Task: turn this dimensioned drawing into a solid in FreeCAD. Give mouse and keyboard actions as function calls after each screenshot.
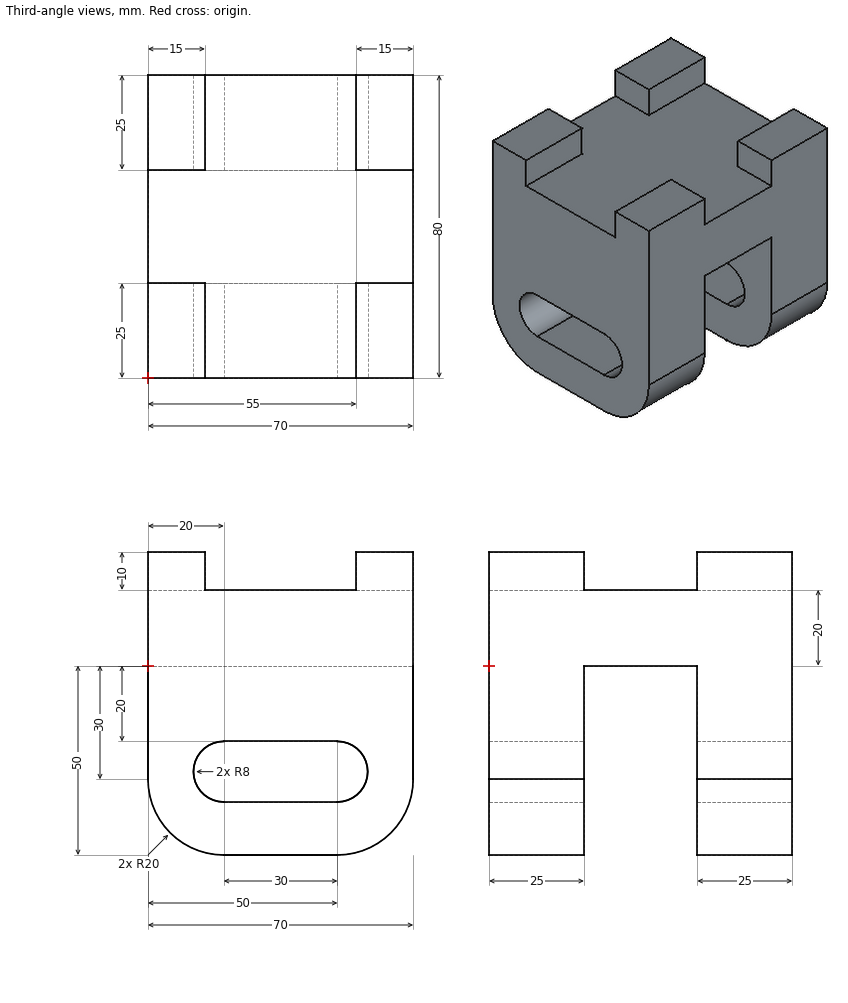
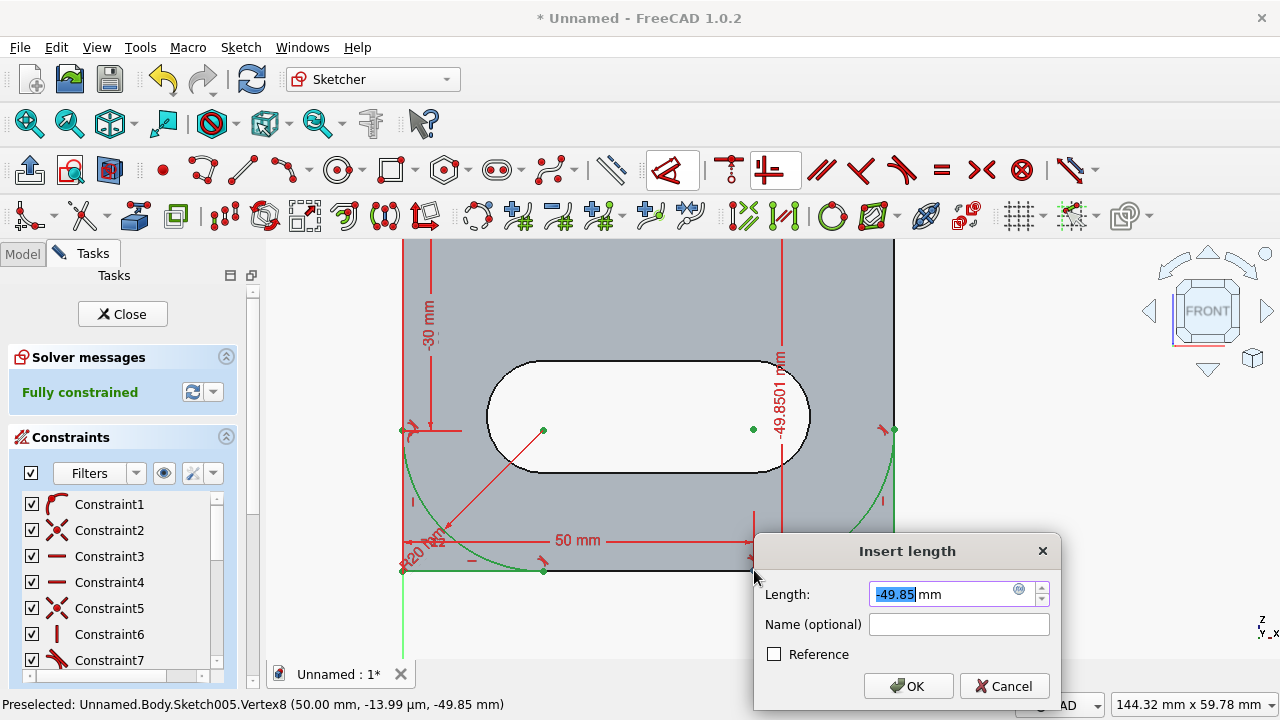
text(-50)
key(Return)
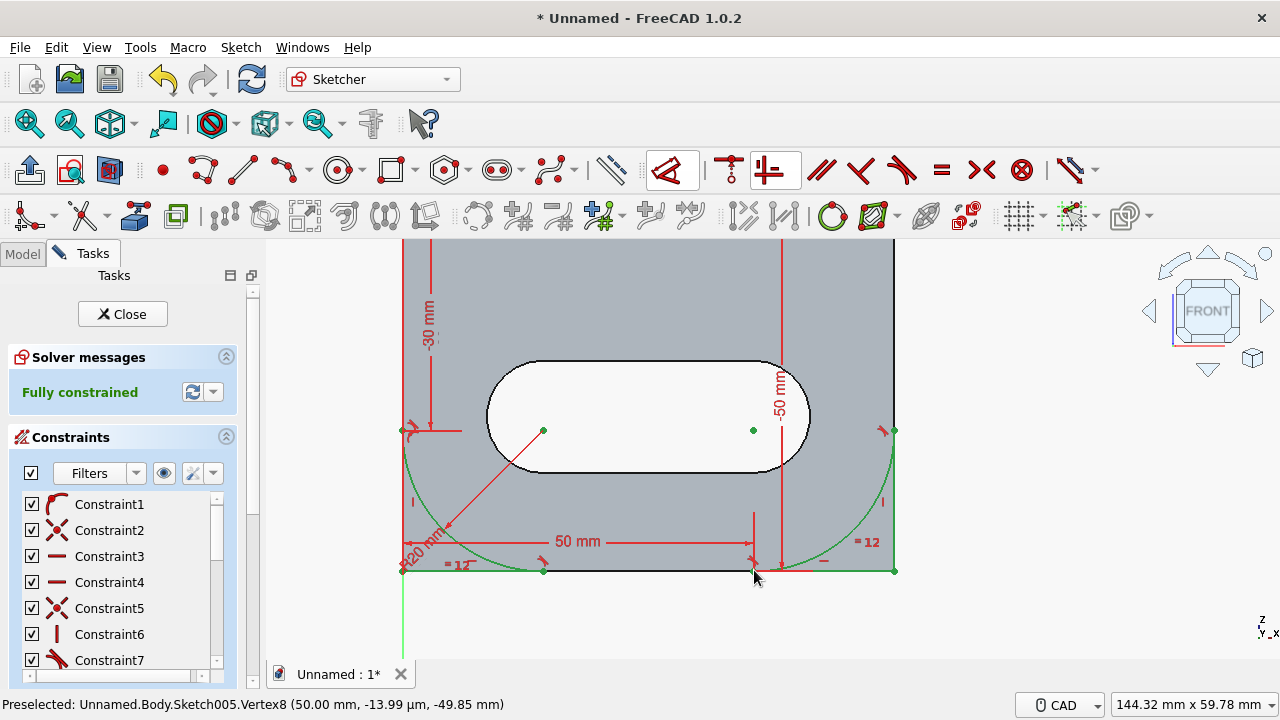
click(123, 314)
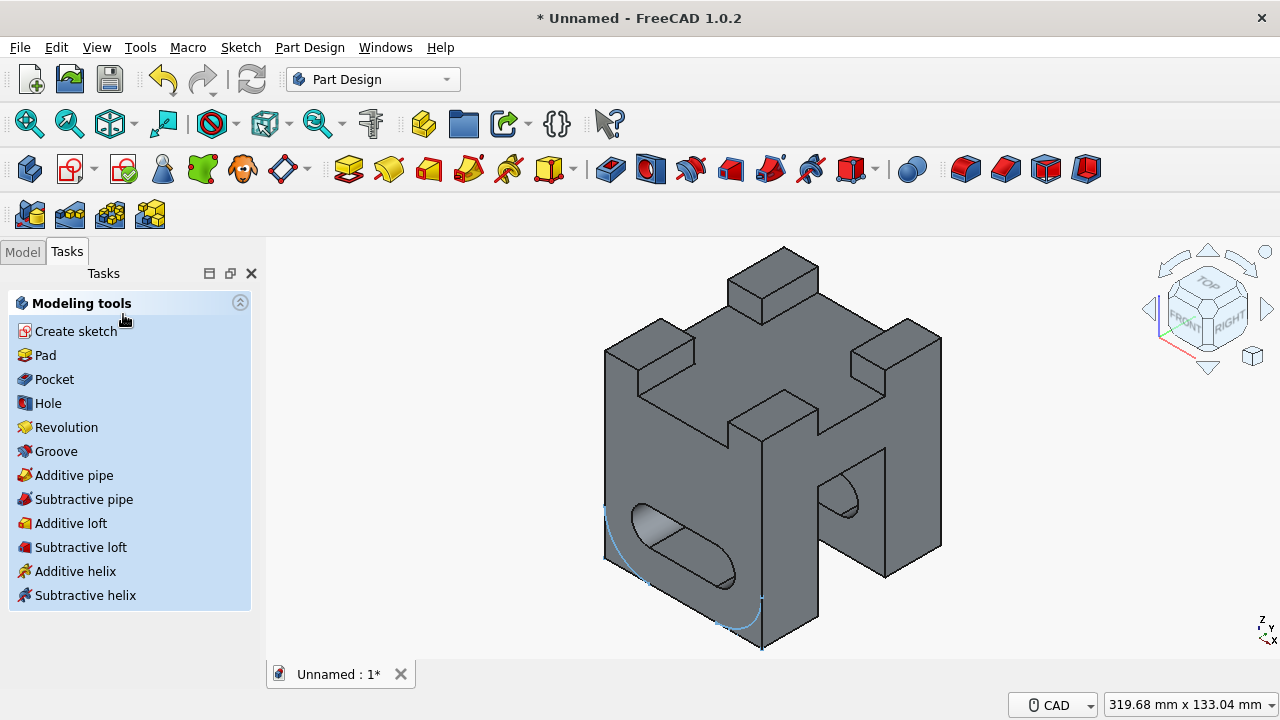
click(612, 170)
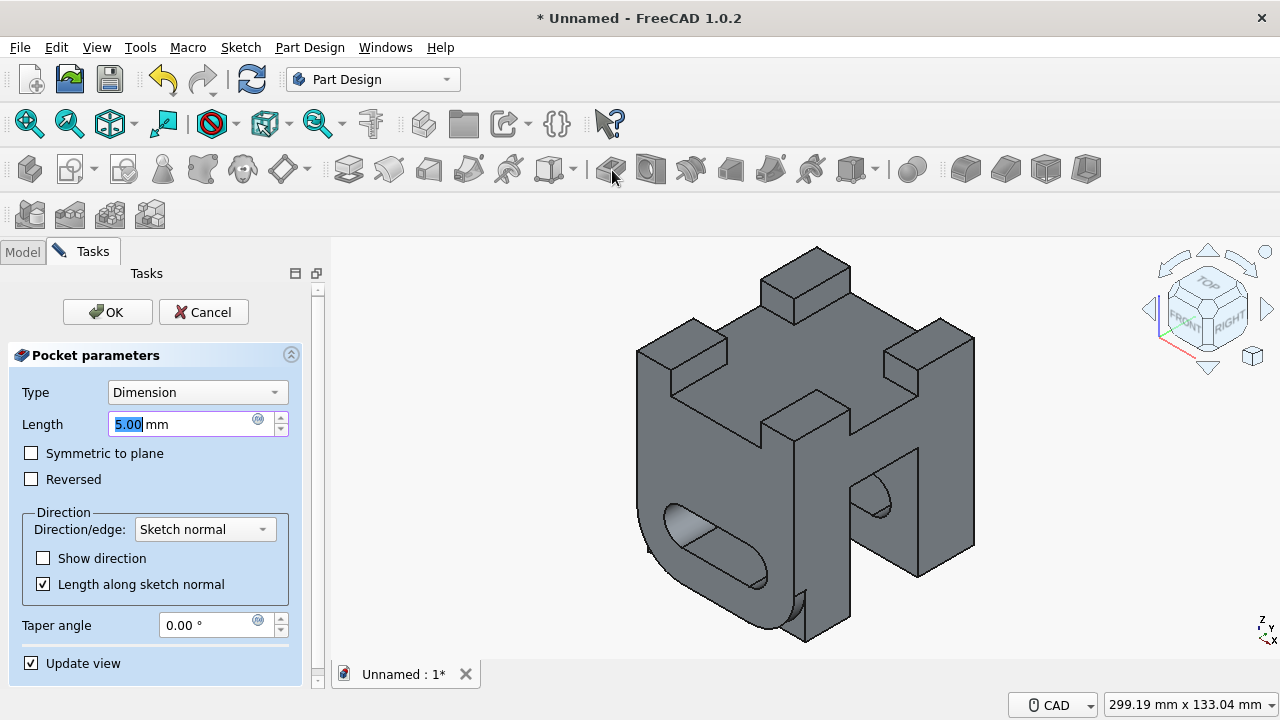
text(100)
key(Tab)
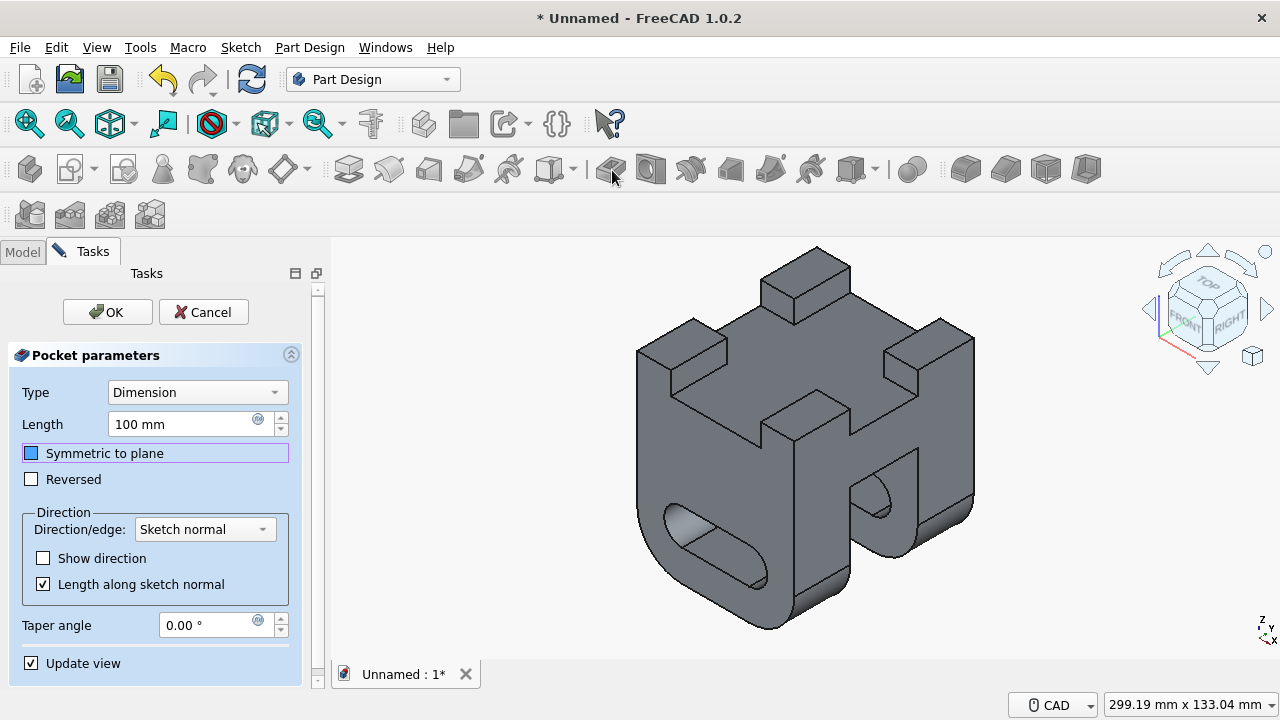
click(108, 312)